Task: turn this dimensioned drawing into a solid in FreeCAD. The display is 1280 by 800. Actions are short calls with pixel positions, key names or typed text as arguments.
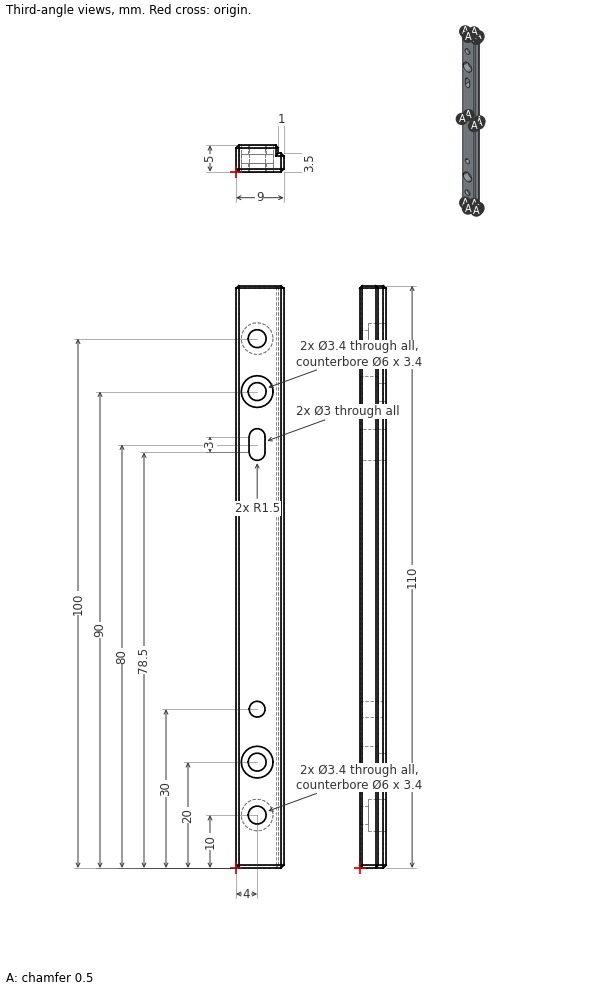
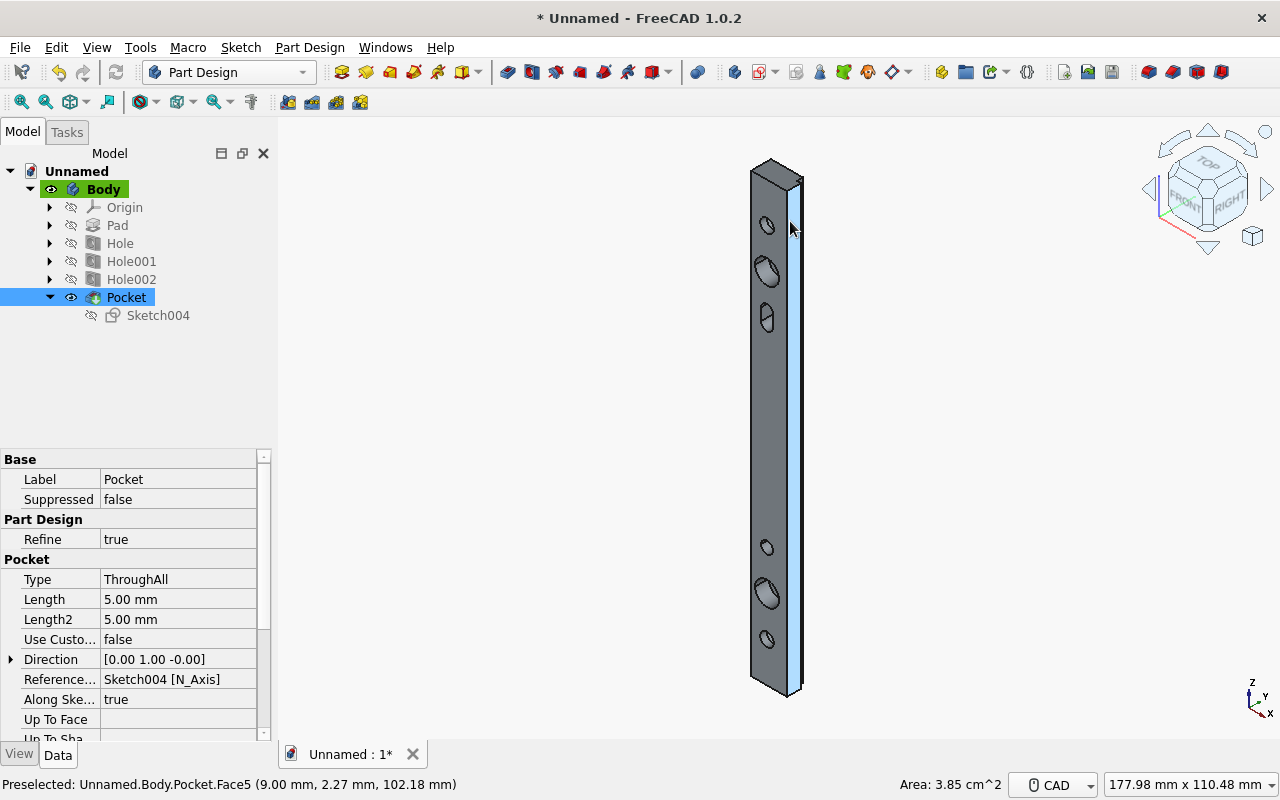
click(779, 174, ctrl)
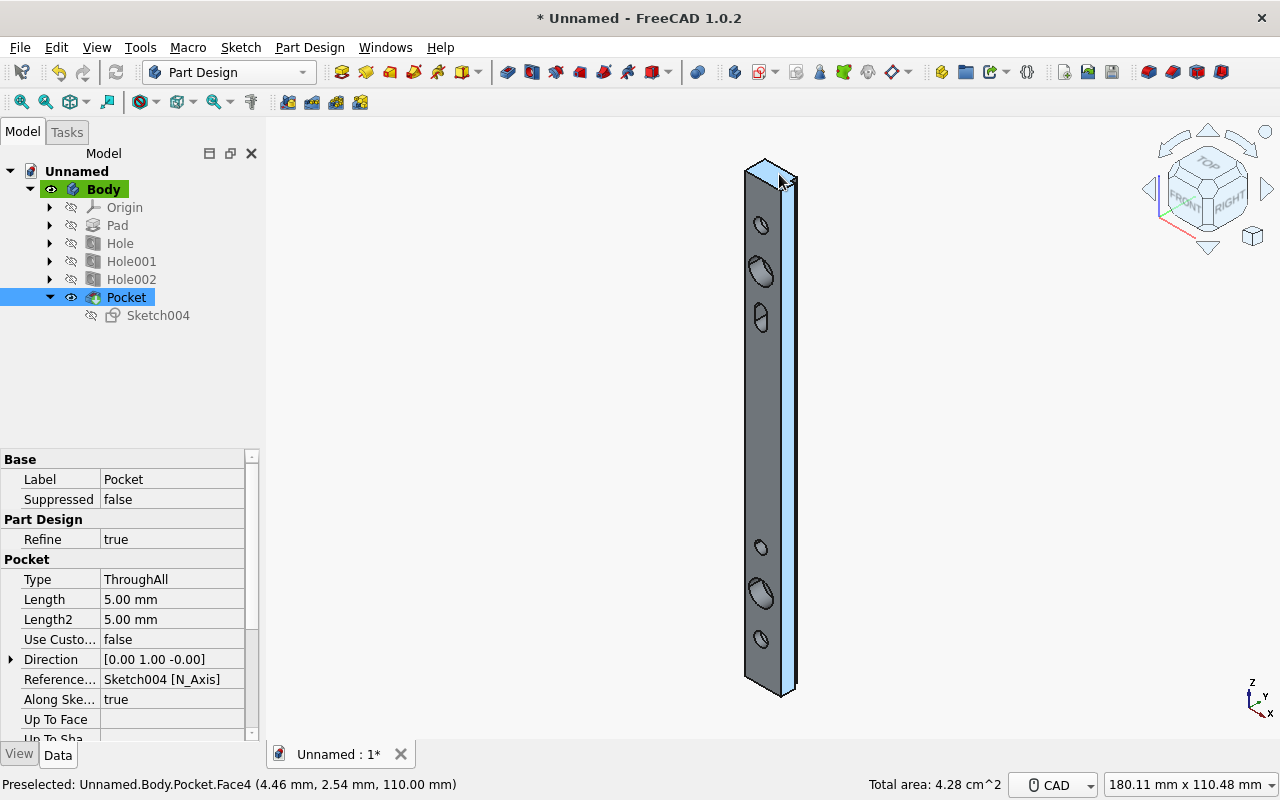
key(2)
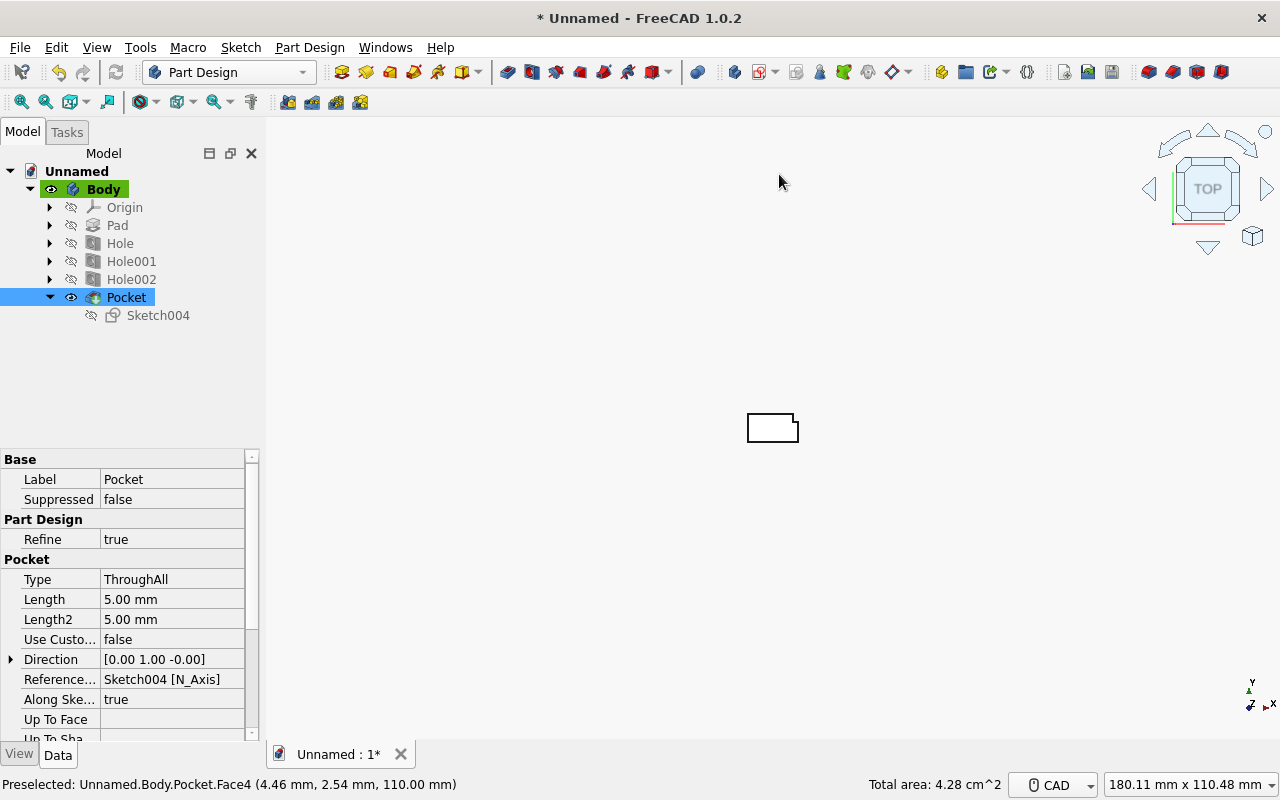
click(22, 102)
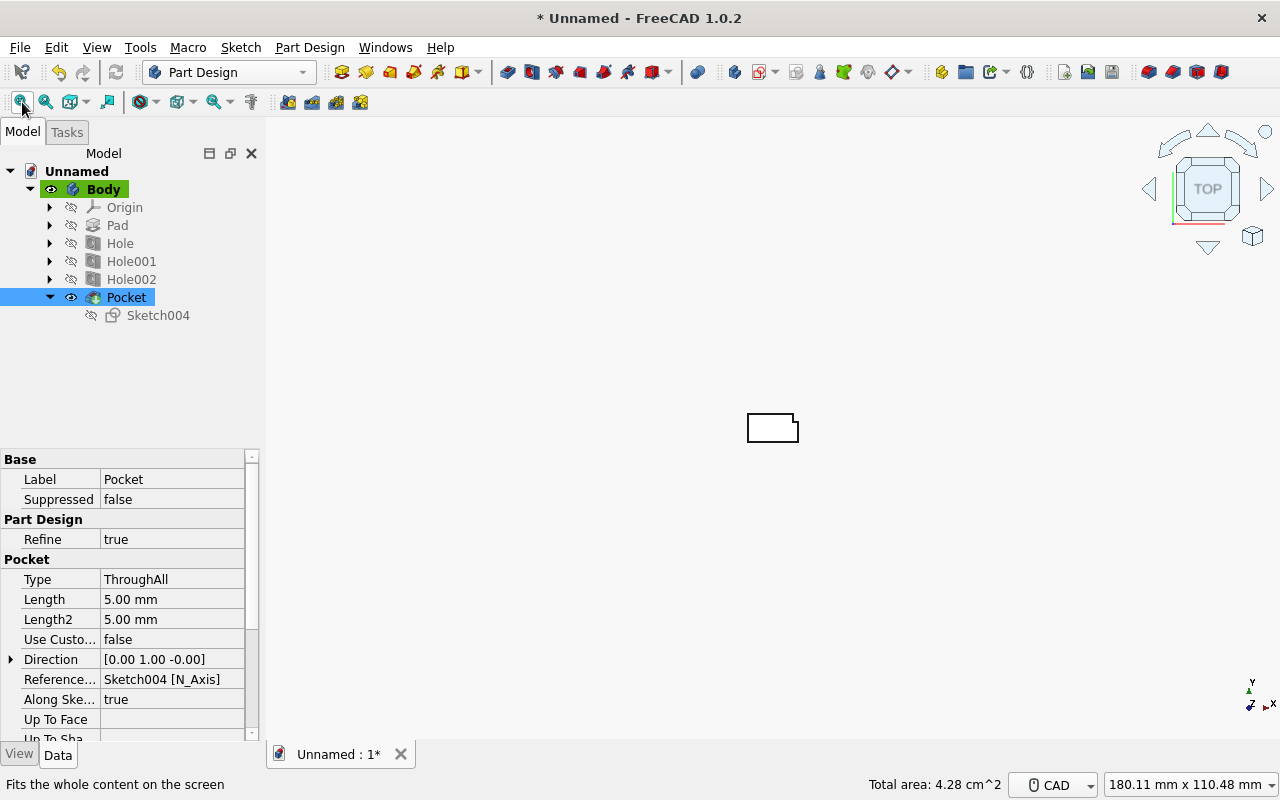
key(0)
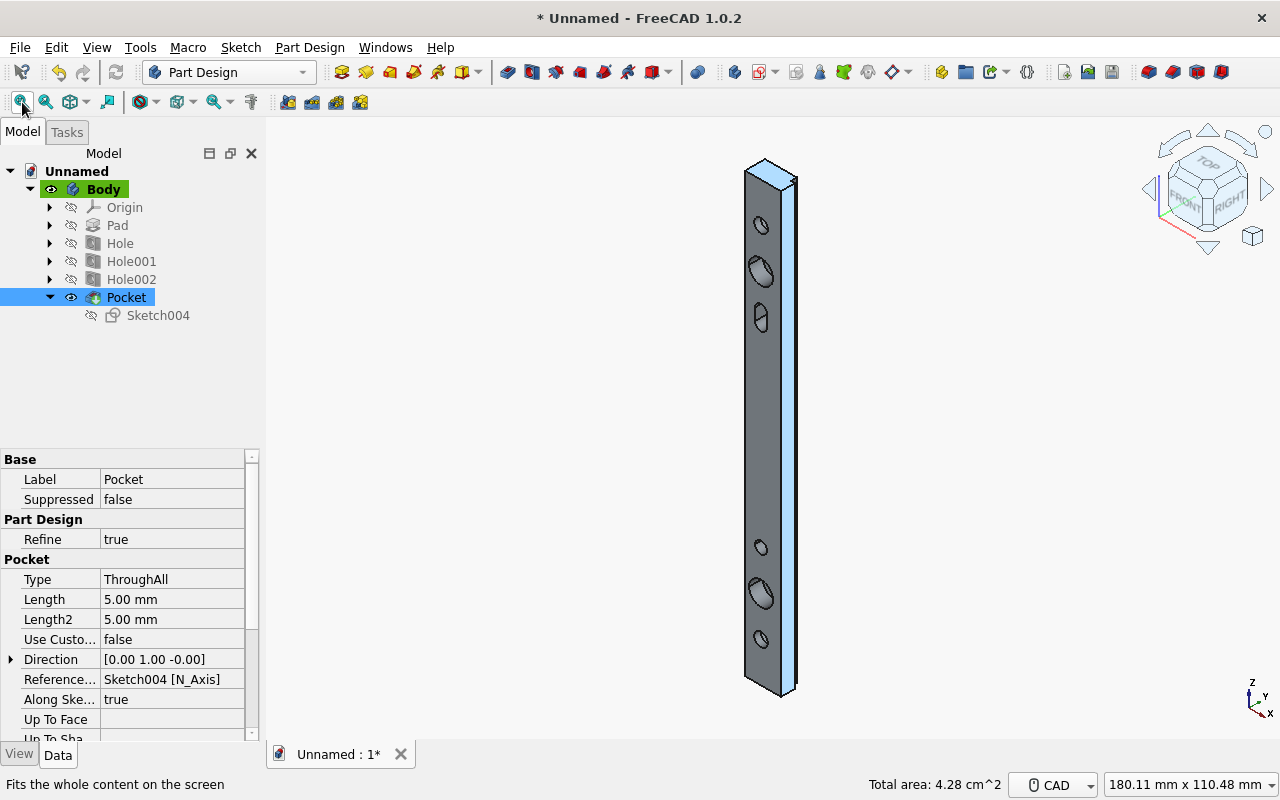
key(1)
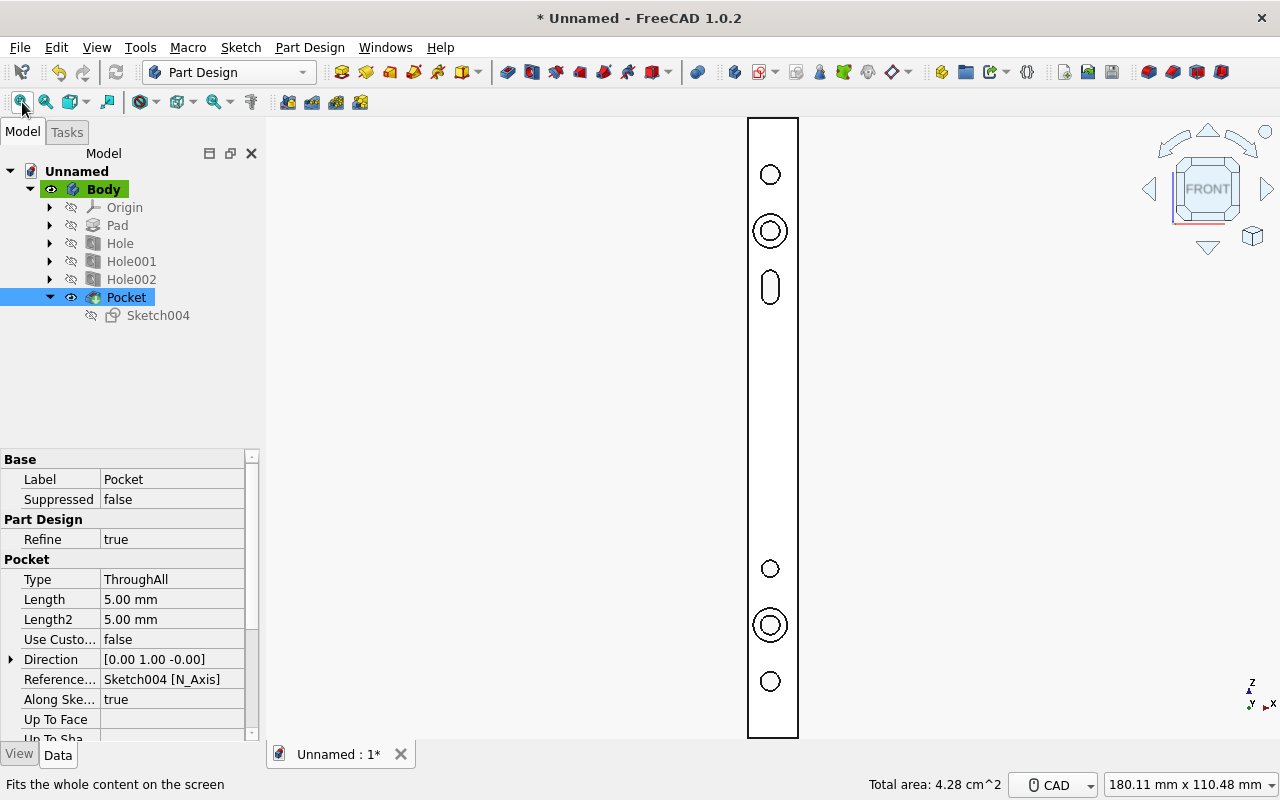
key(3)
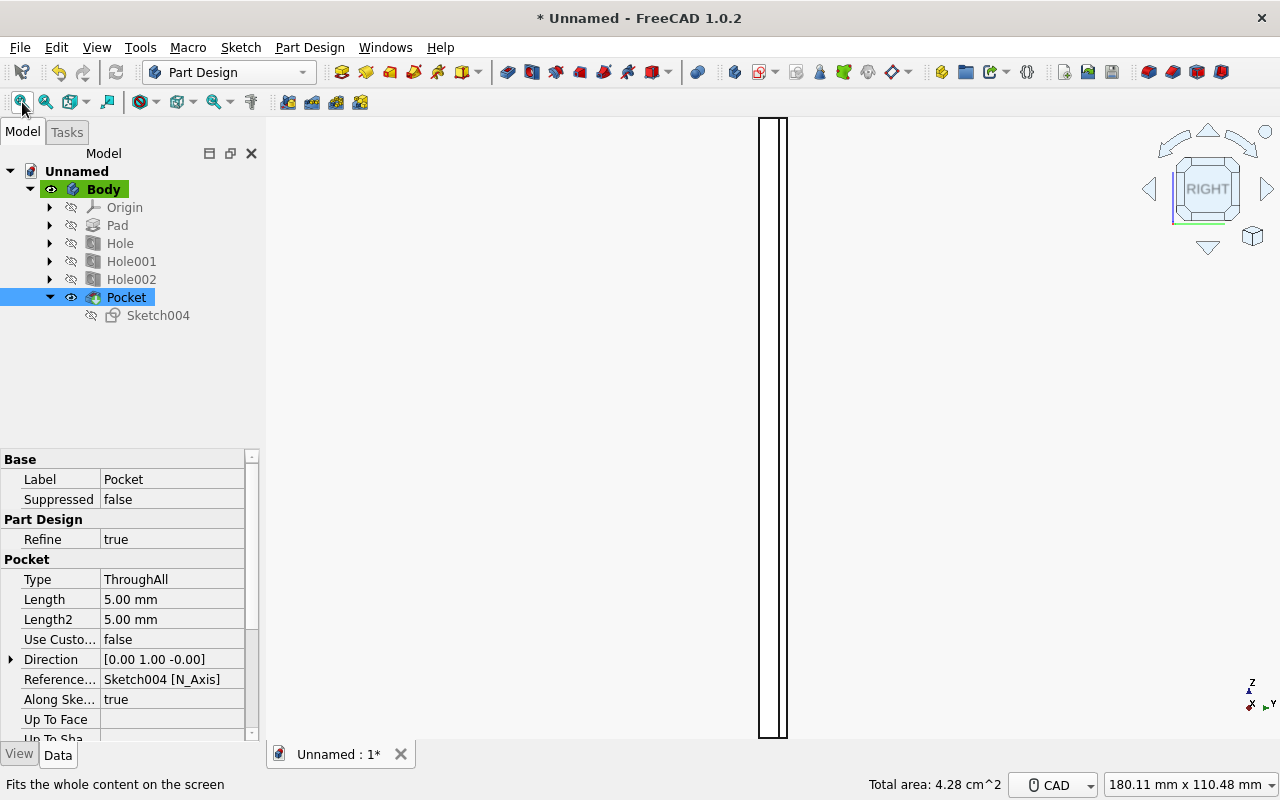
click(787, 427, ctrl)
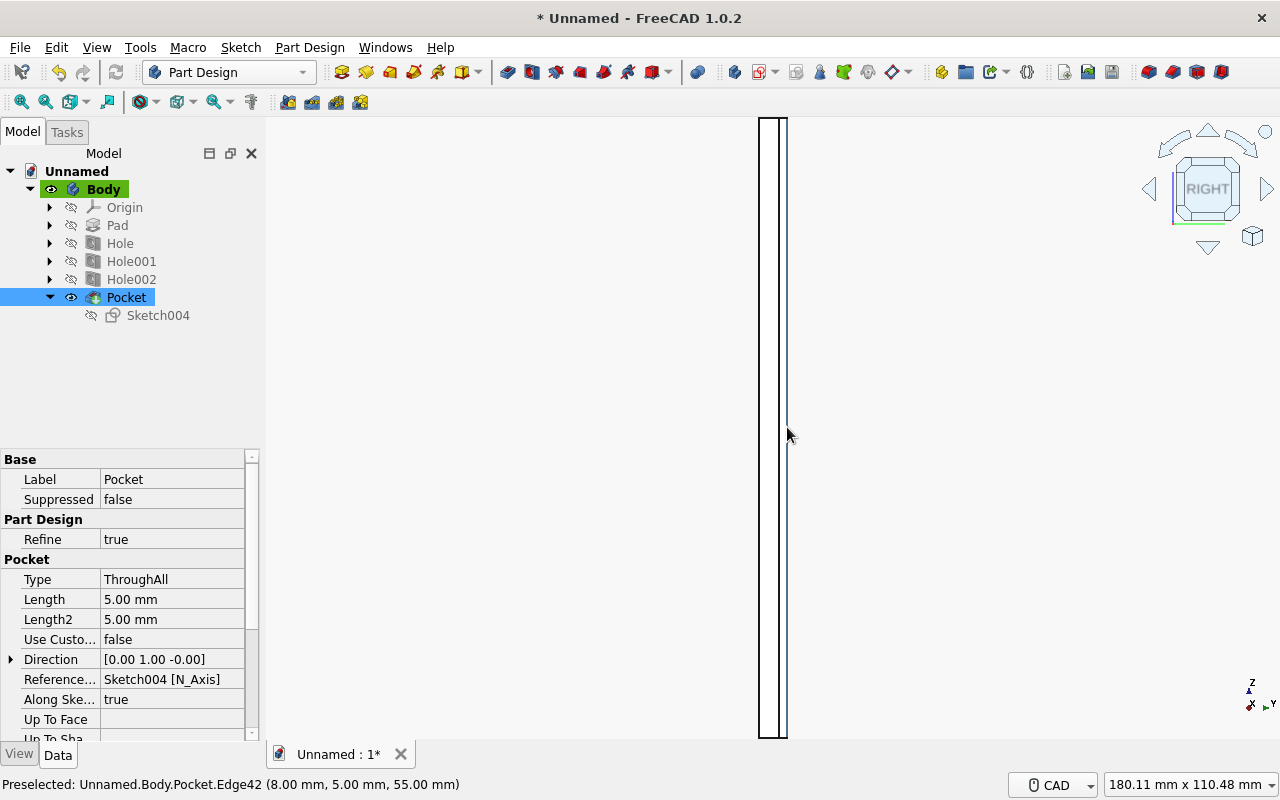
key(5)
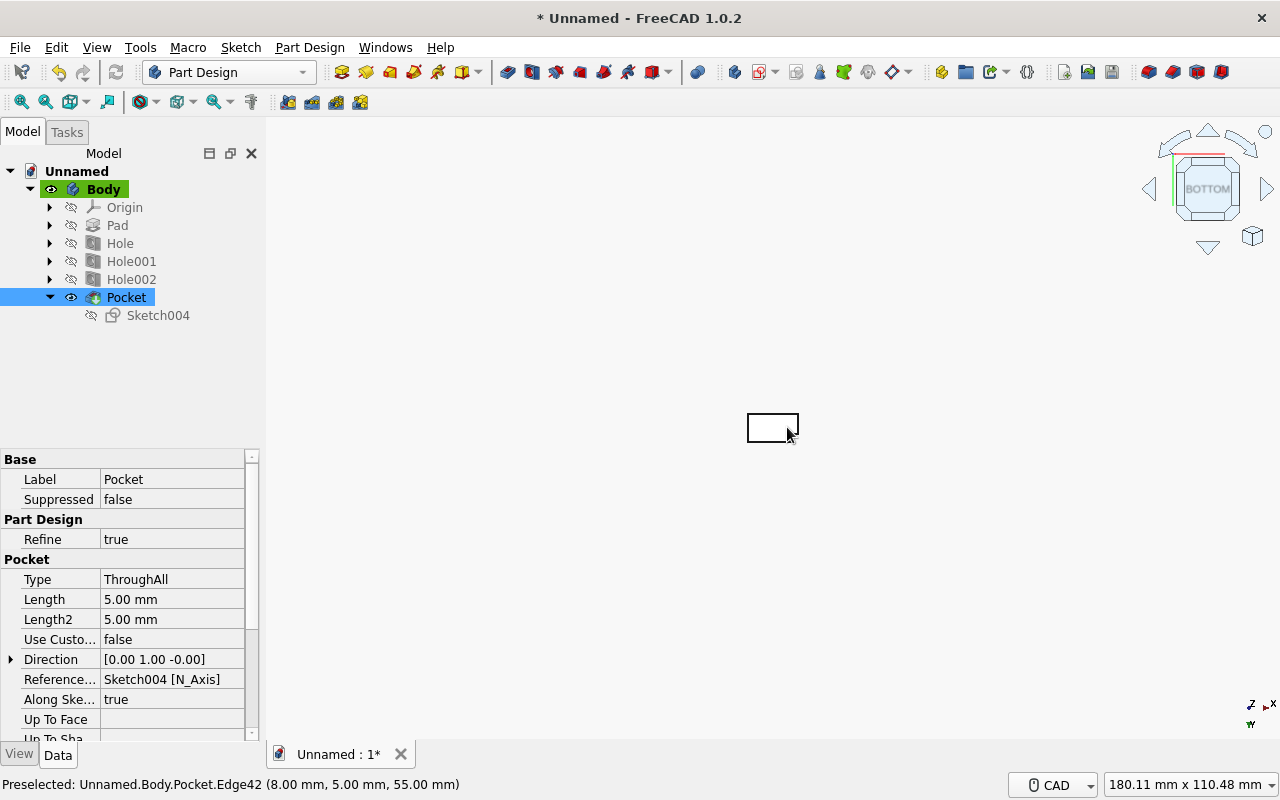
click(22, 102)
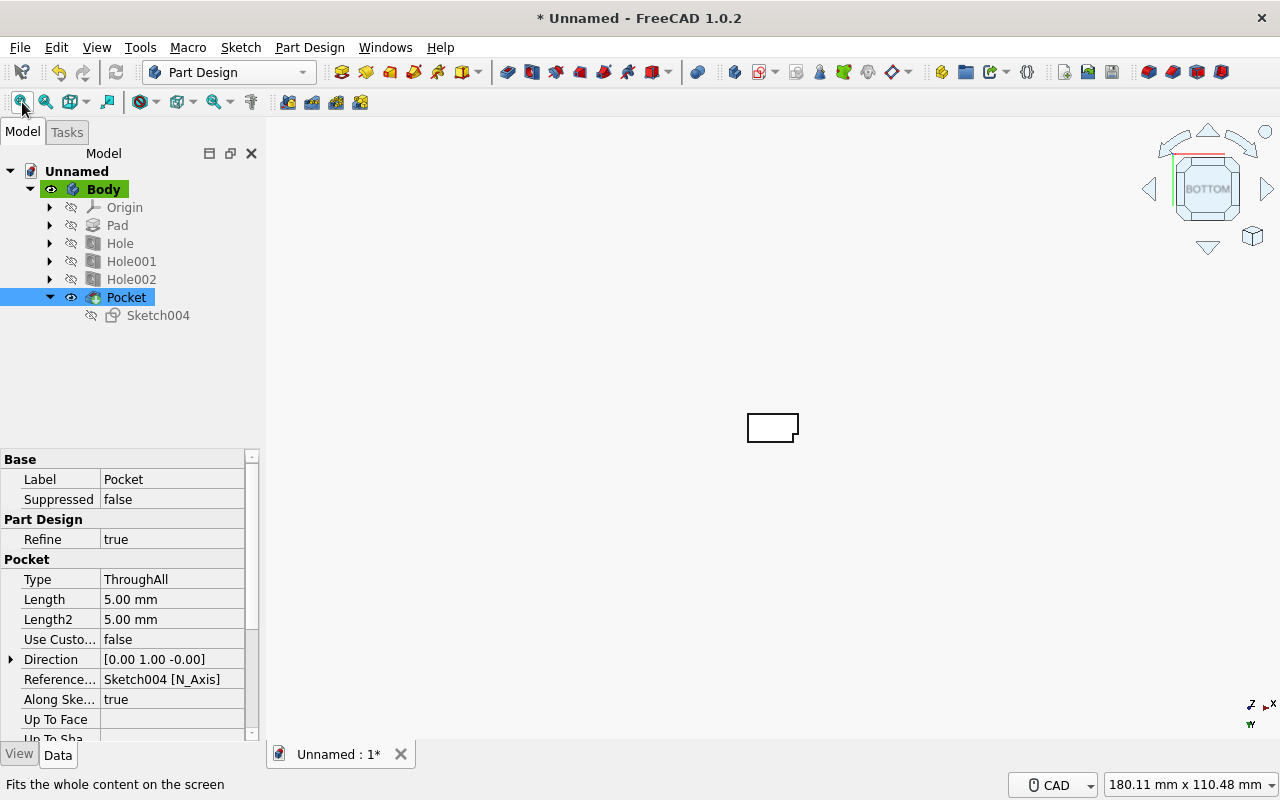
click(773, 427, ctrl)